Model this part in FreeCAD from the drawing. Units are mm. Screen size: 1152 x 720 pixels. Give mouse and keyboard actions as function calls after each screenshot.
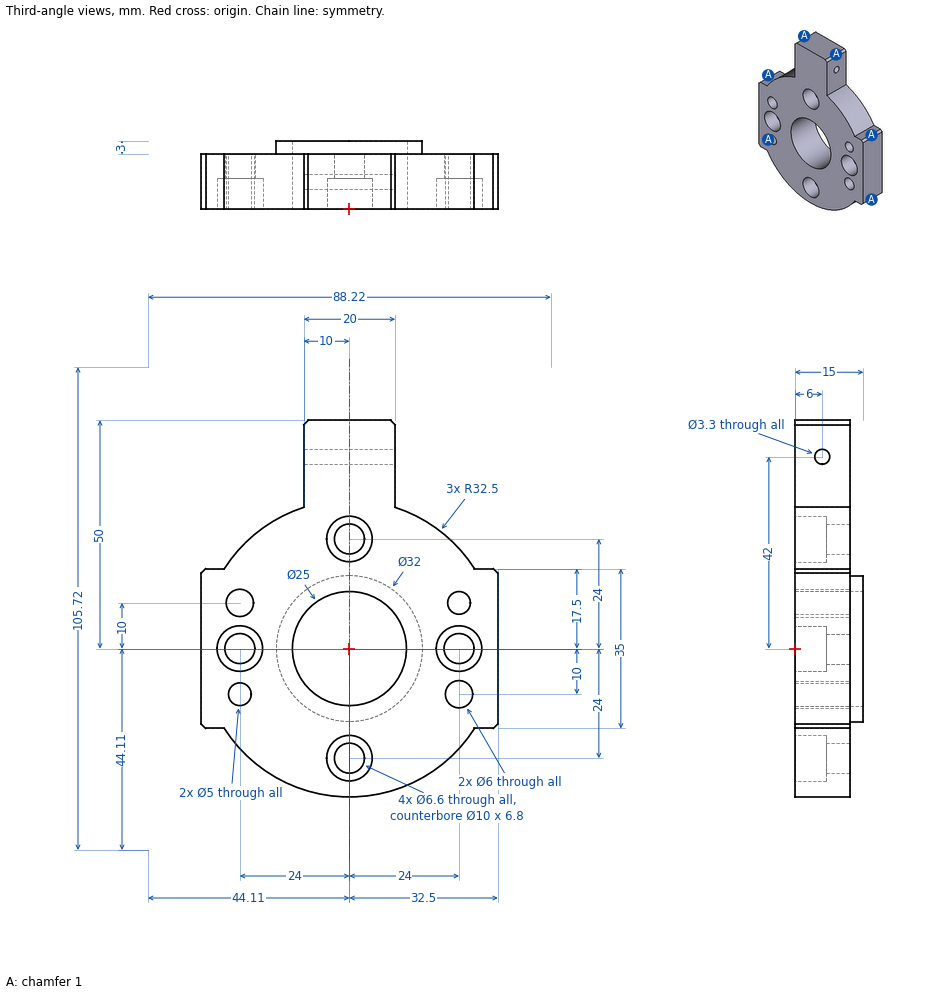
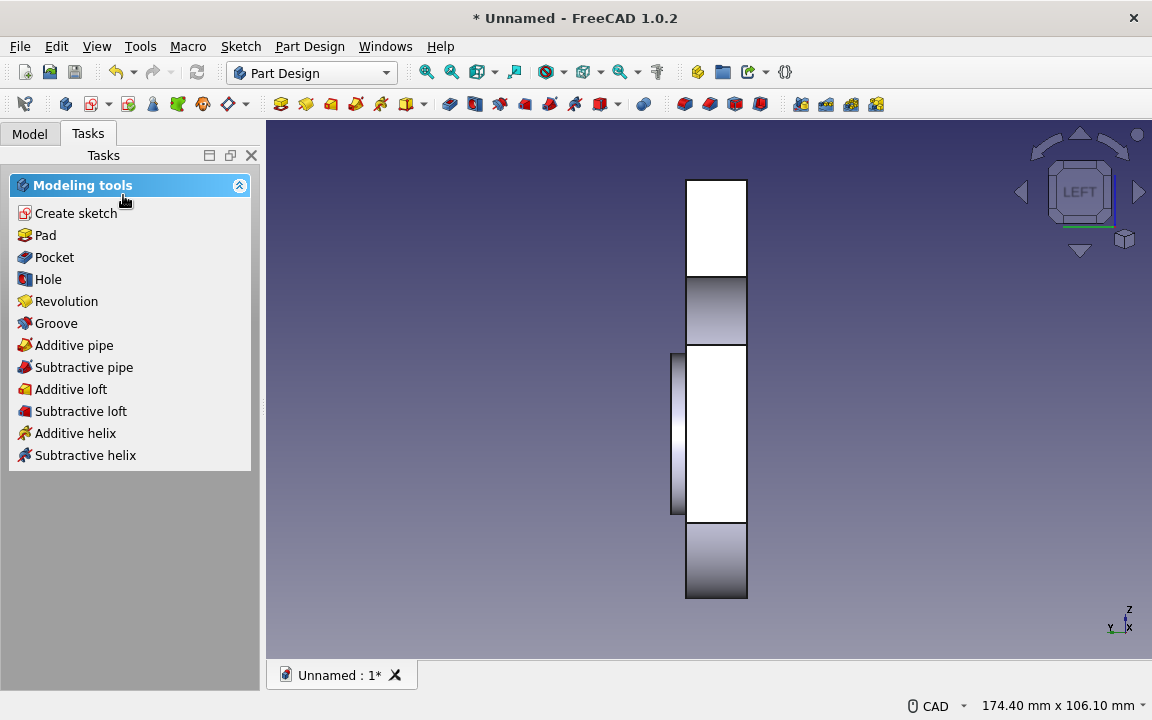
click(475, 104)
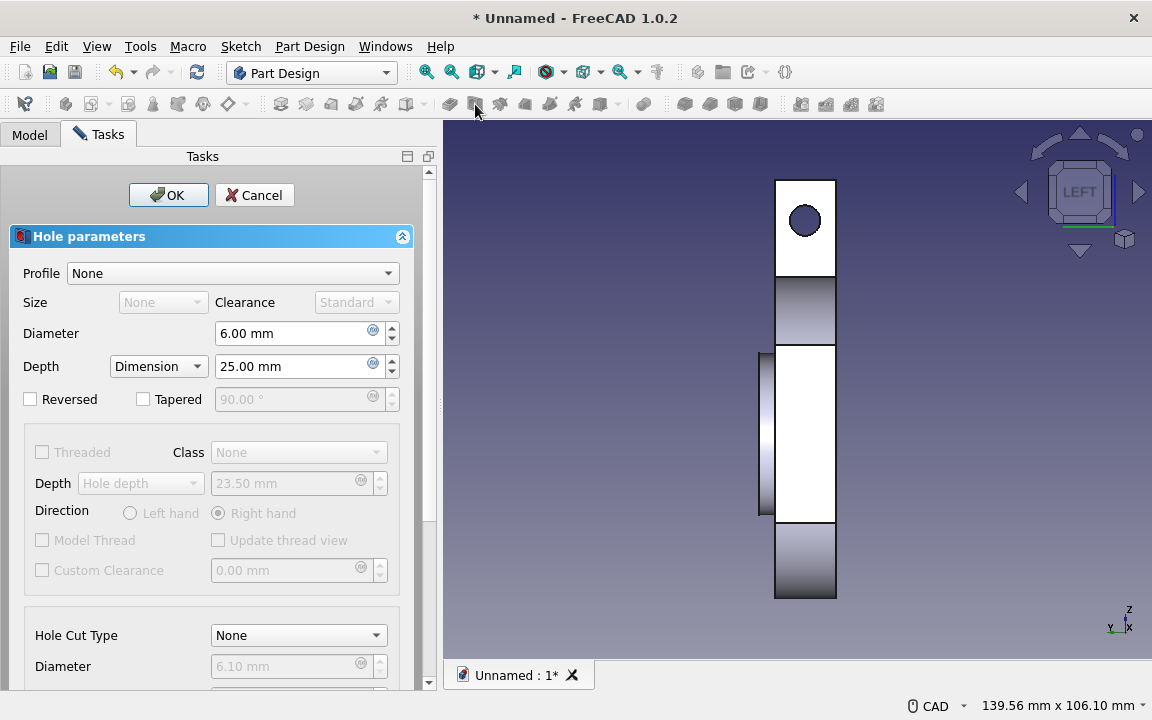
triple_click(300, 334)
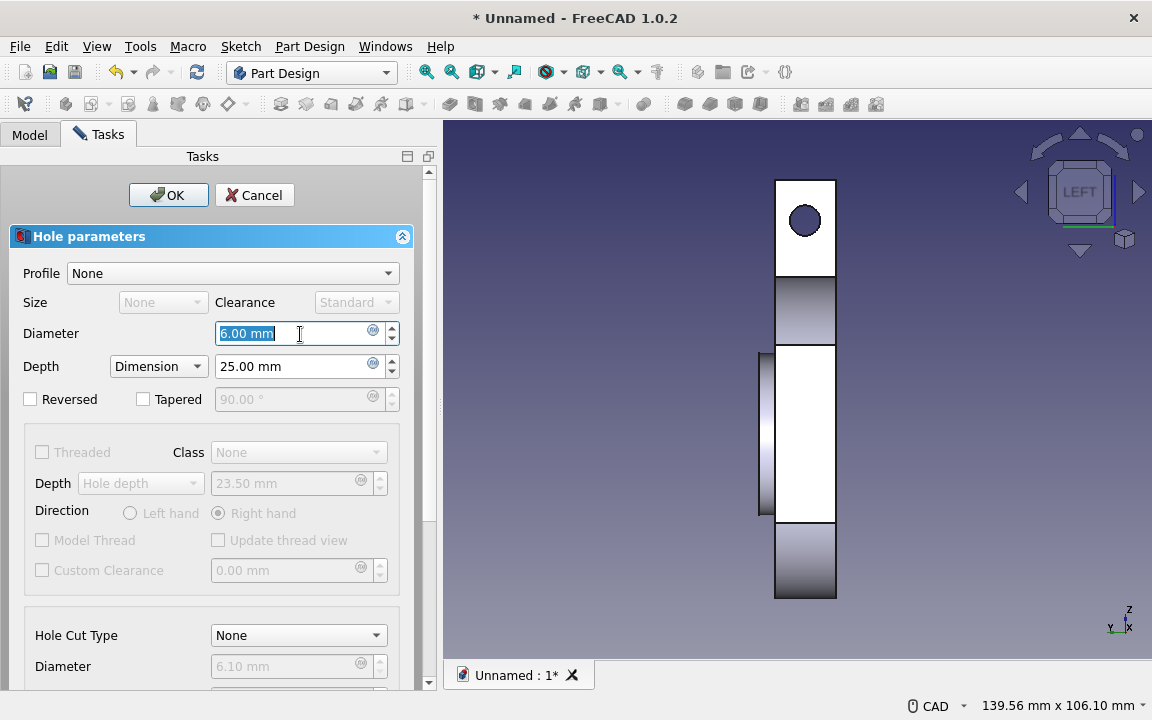
text(3.3)
key(Tab)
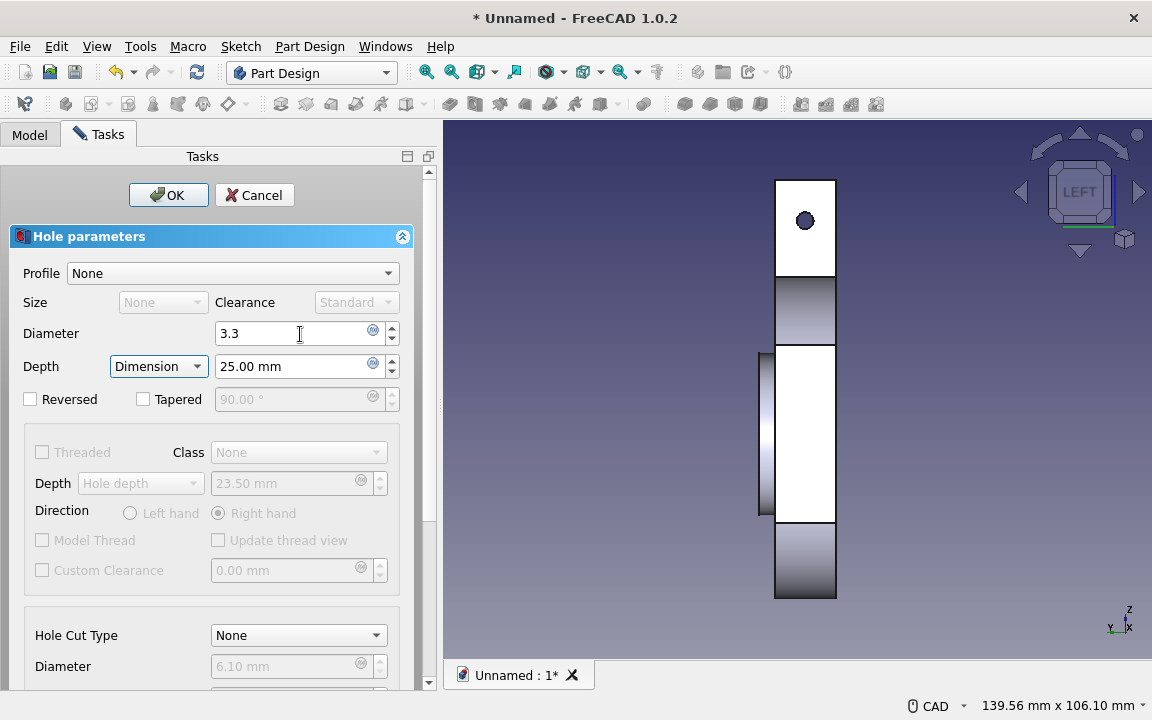
click(160, 366)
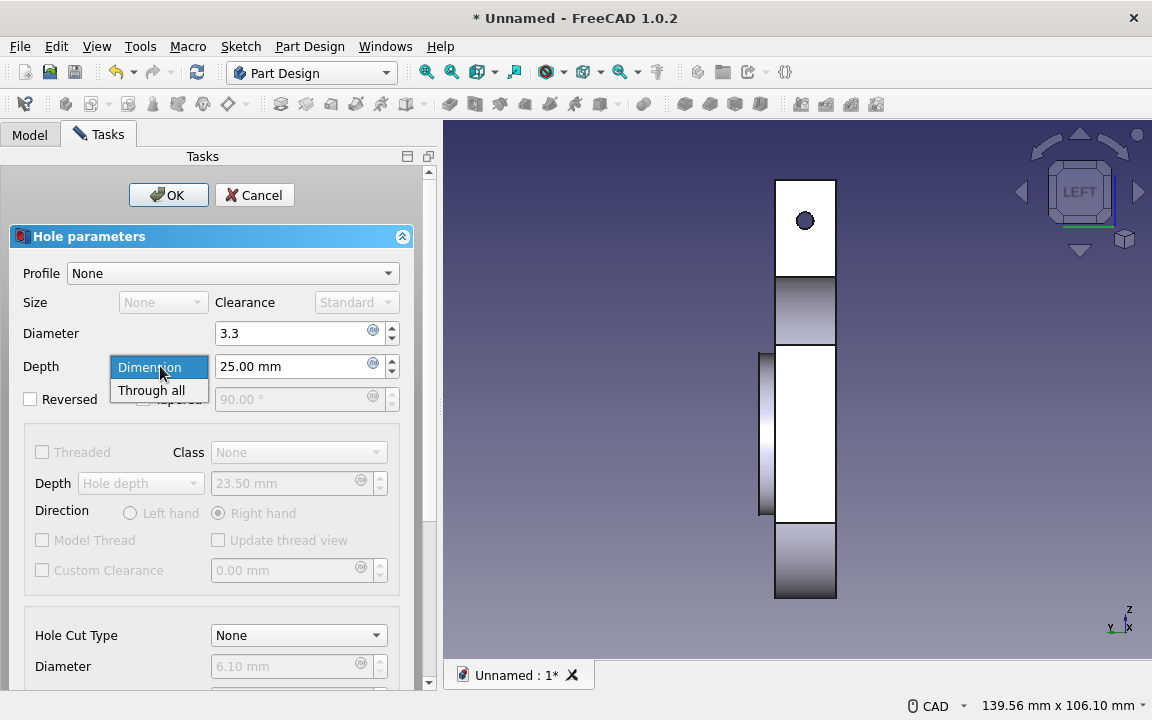
click(158, 390)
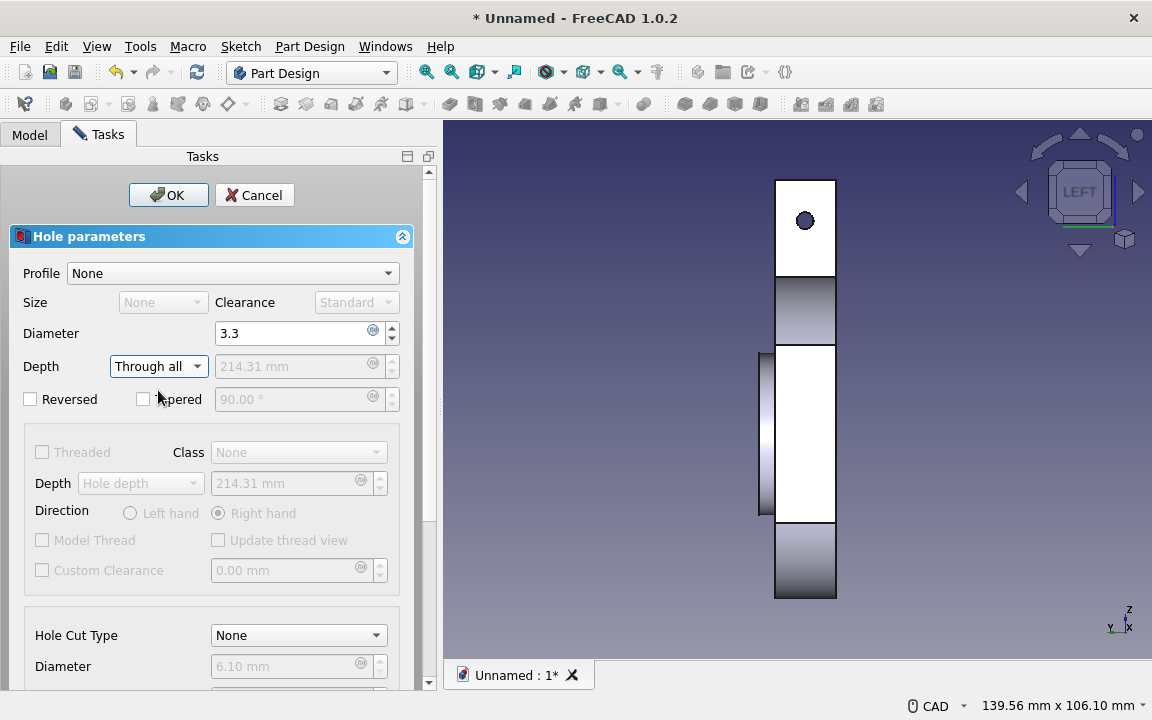
click(169, 195)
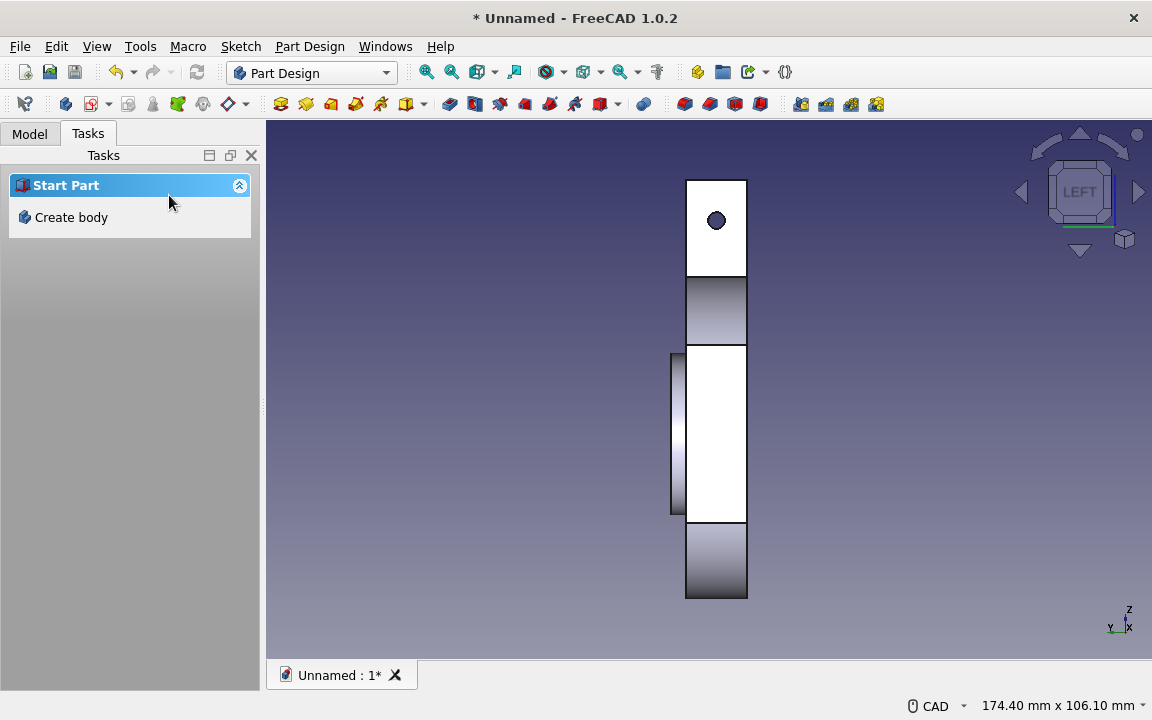
click(90, 104)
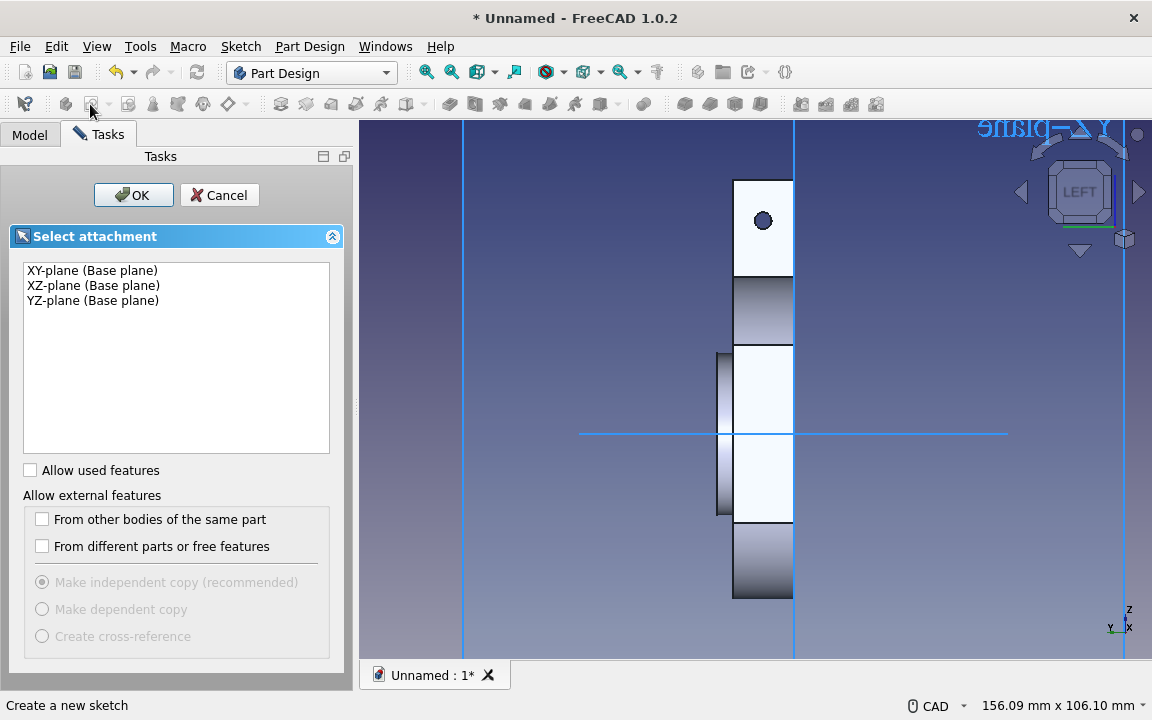
click(84, 286)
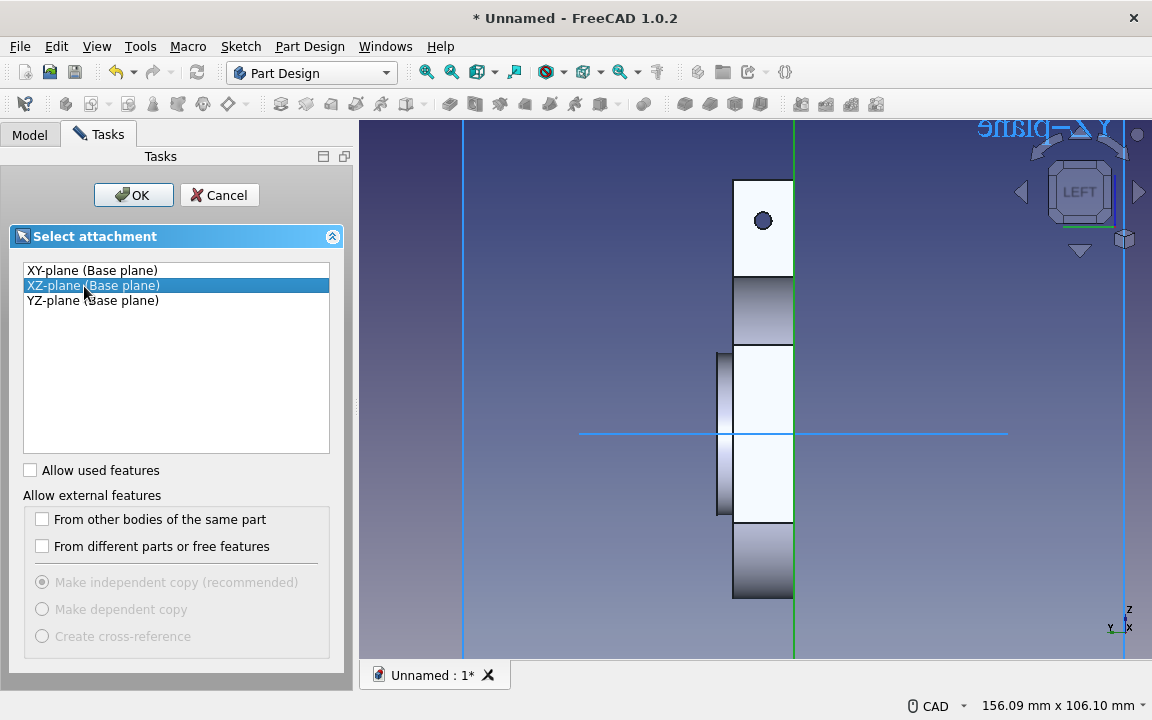
click(134, 195)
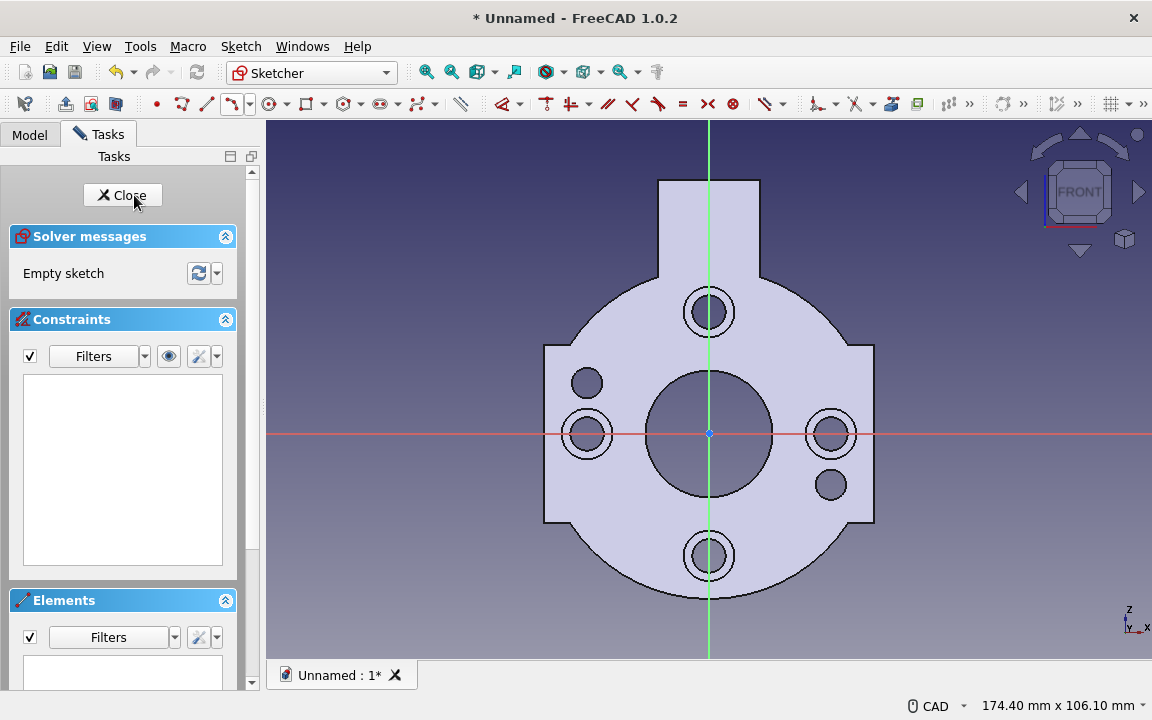
scroll(792, 488, up, 3)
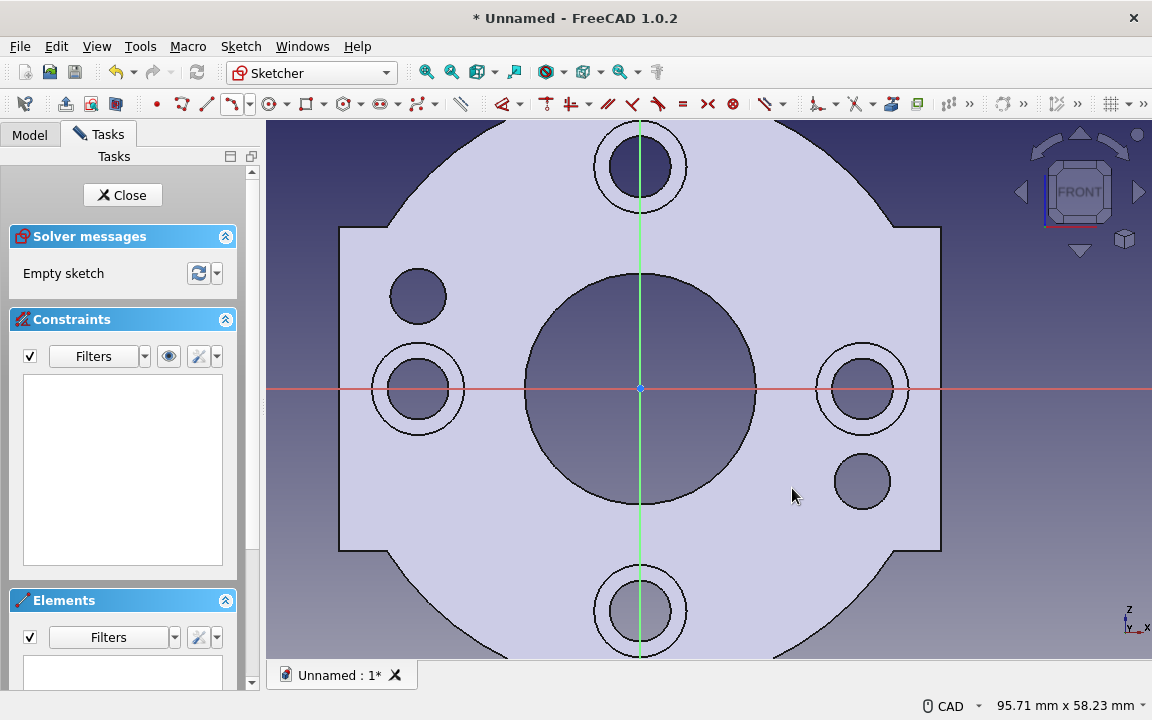
click(268, 104)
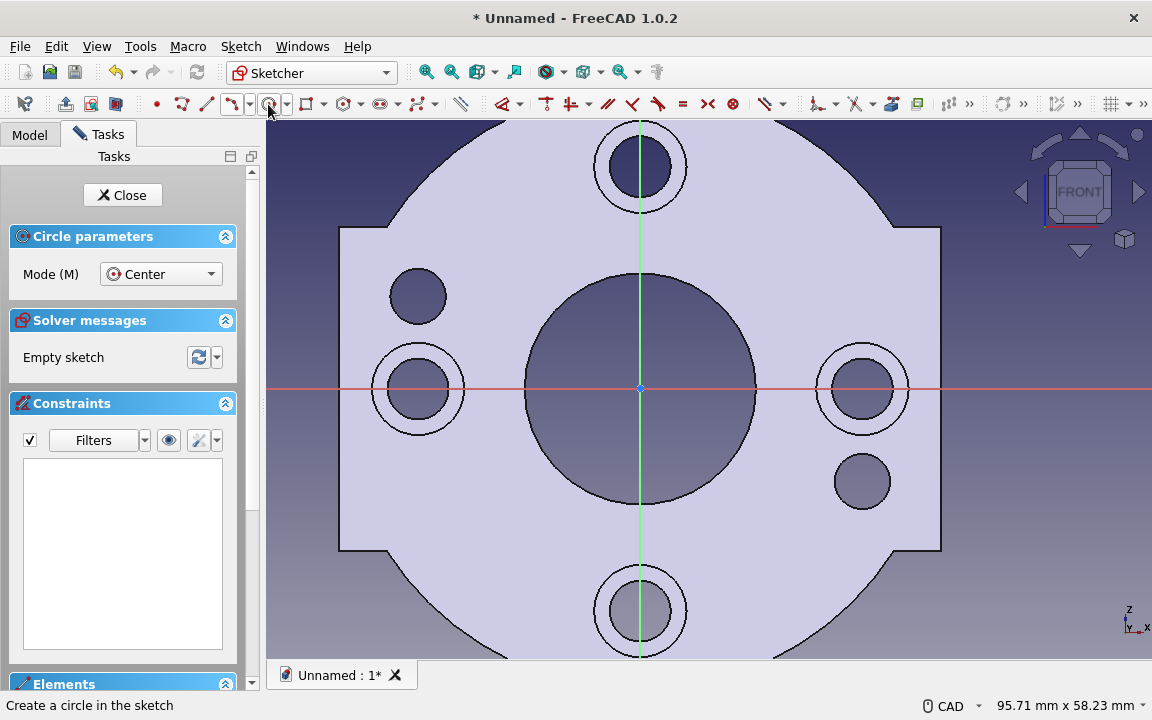
click(418, 482)
click(434, 465)